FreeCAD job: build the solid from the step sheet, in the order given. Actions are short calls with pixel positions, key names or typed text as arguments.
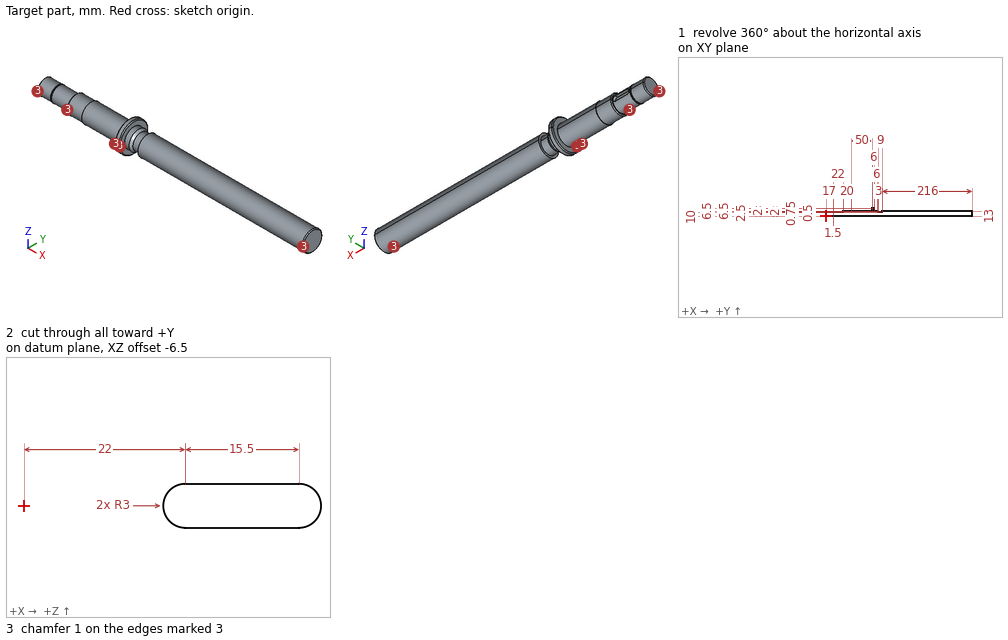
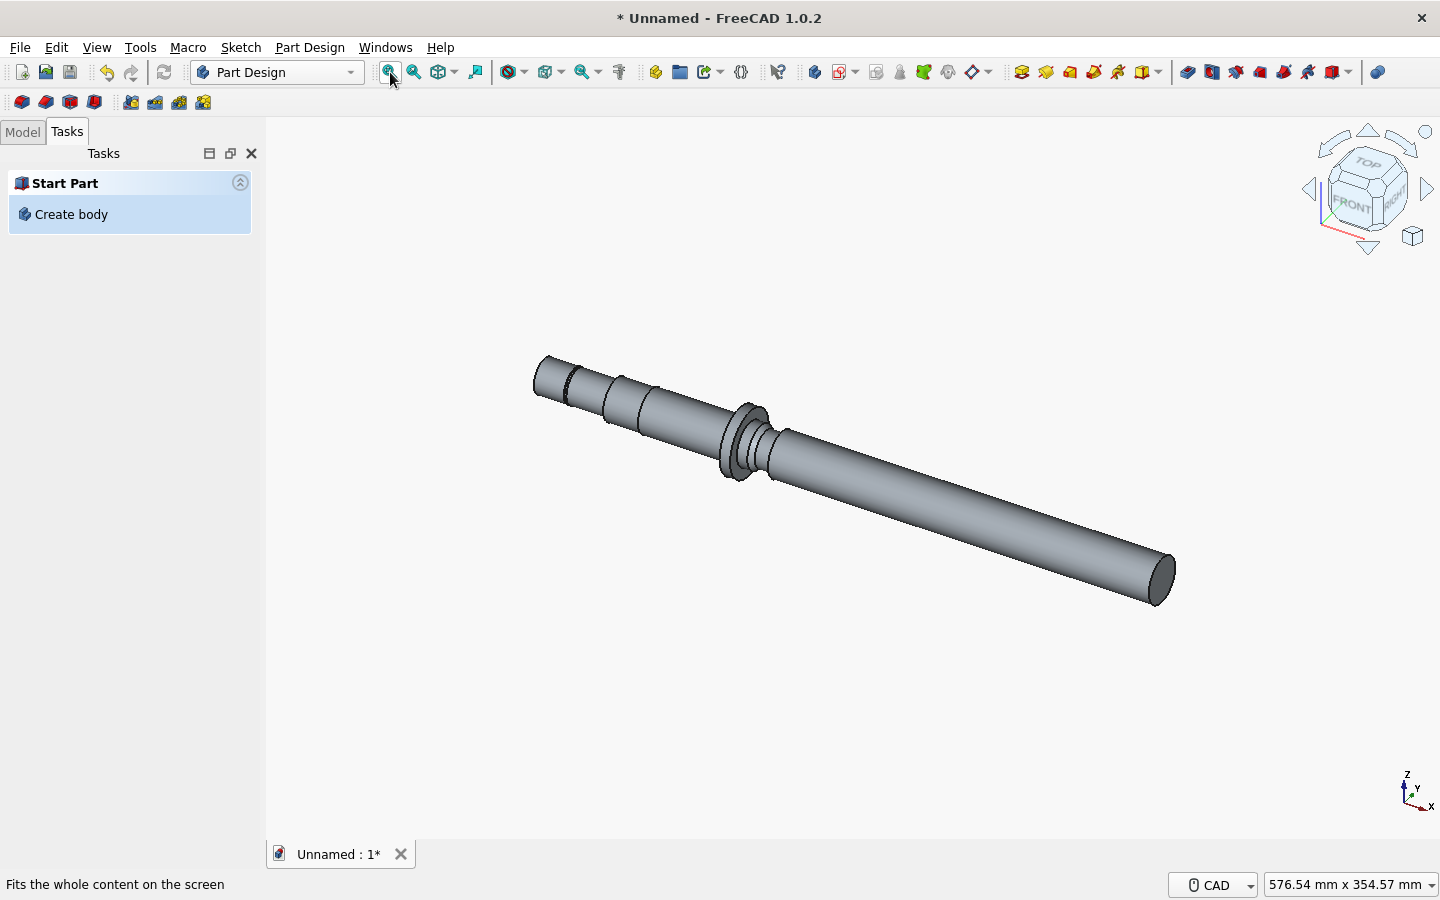
click(23, 131)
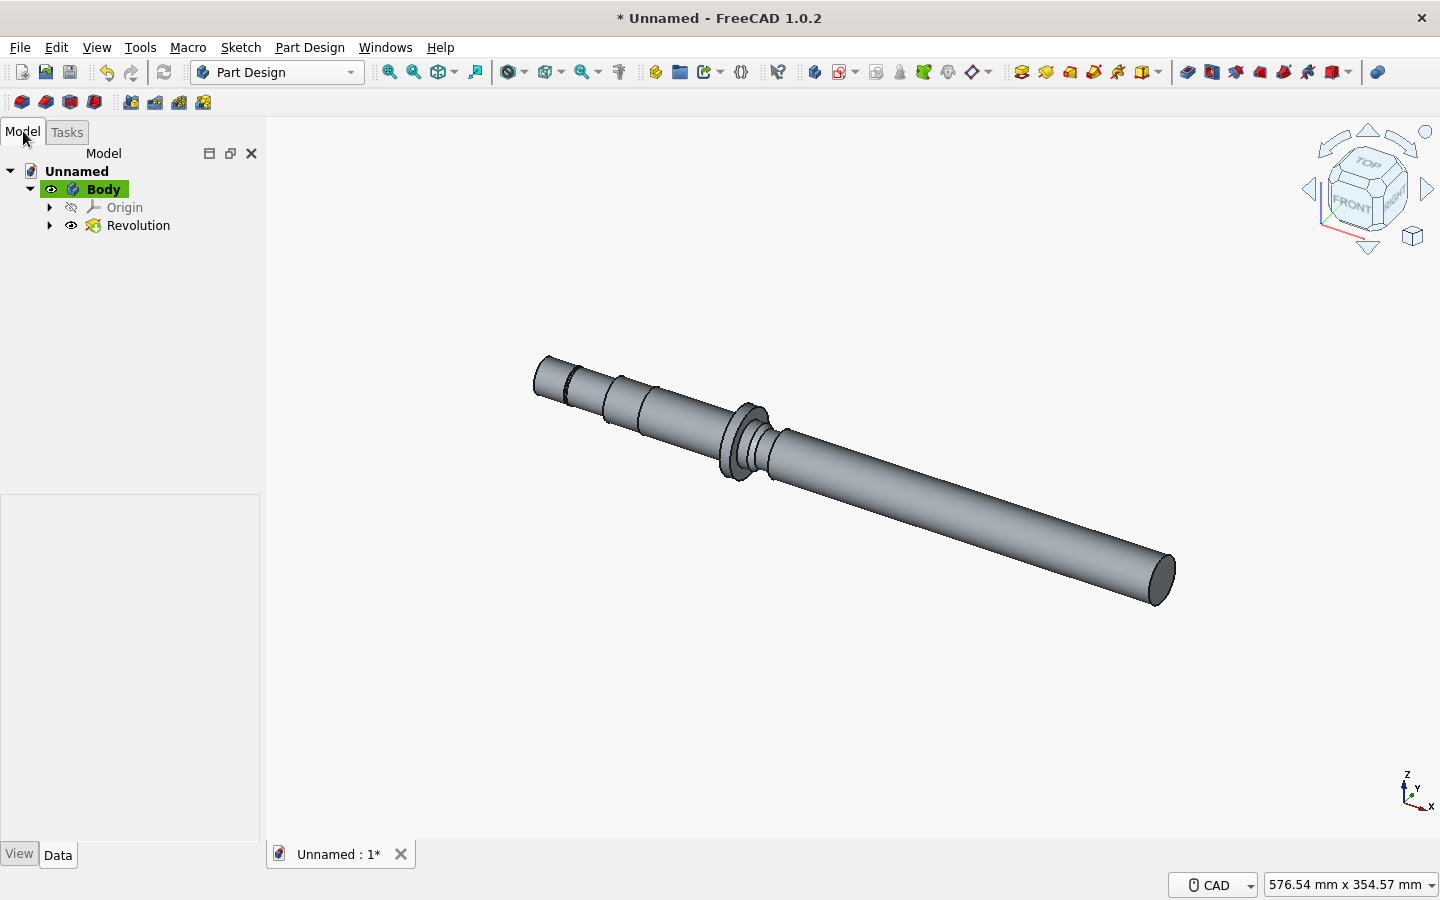
click(50, 207)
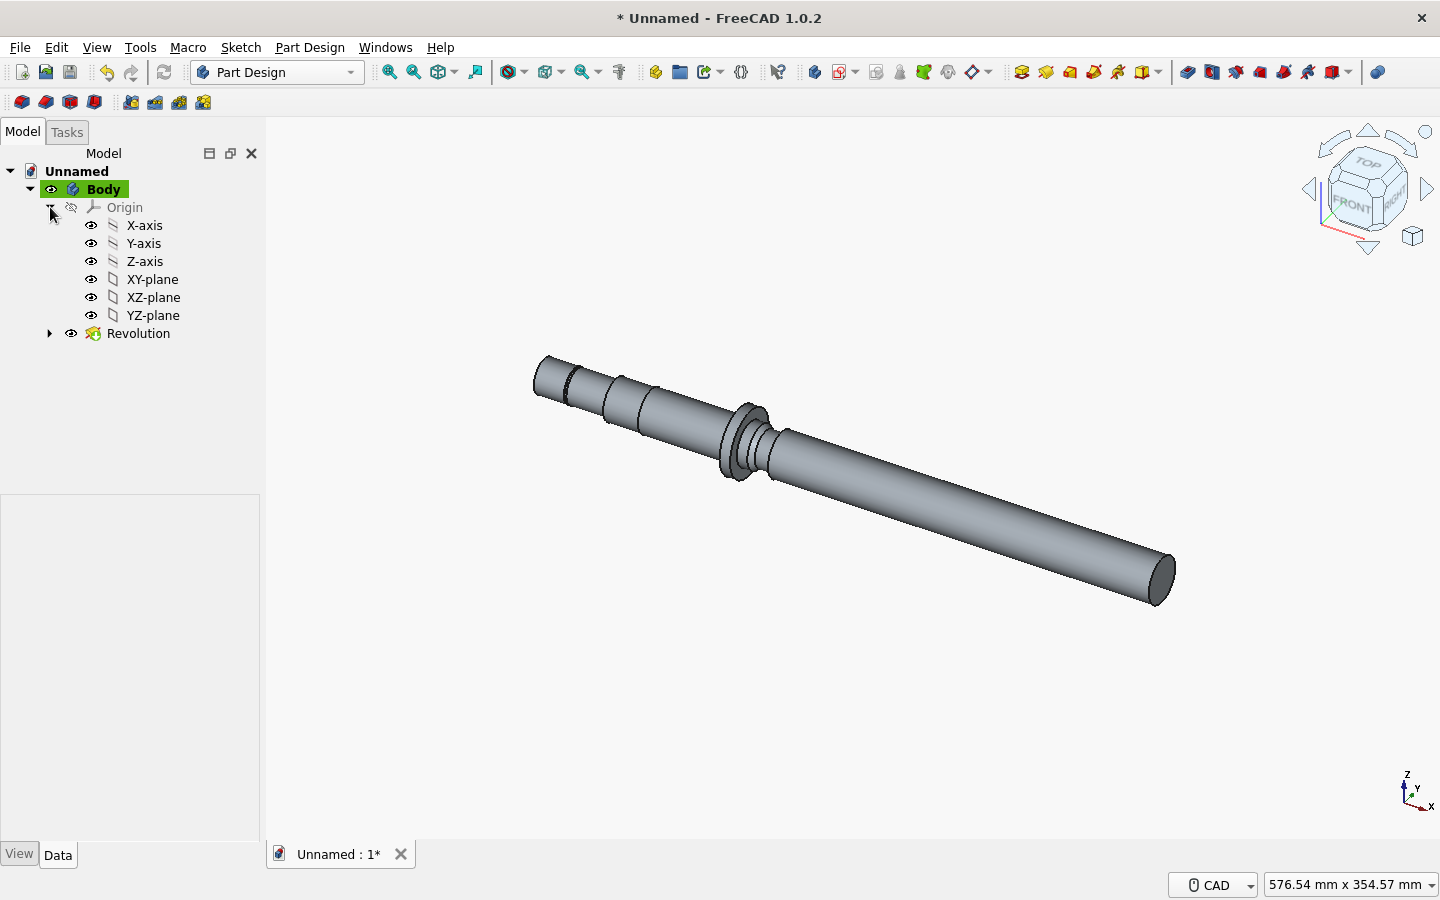
click(136, 297)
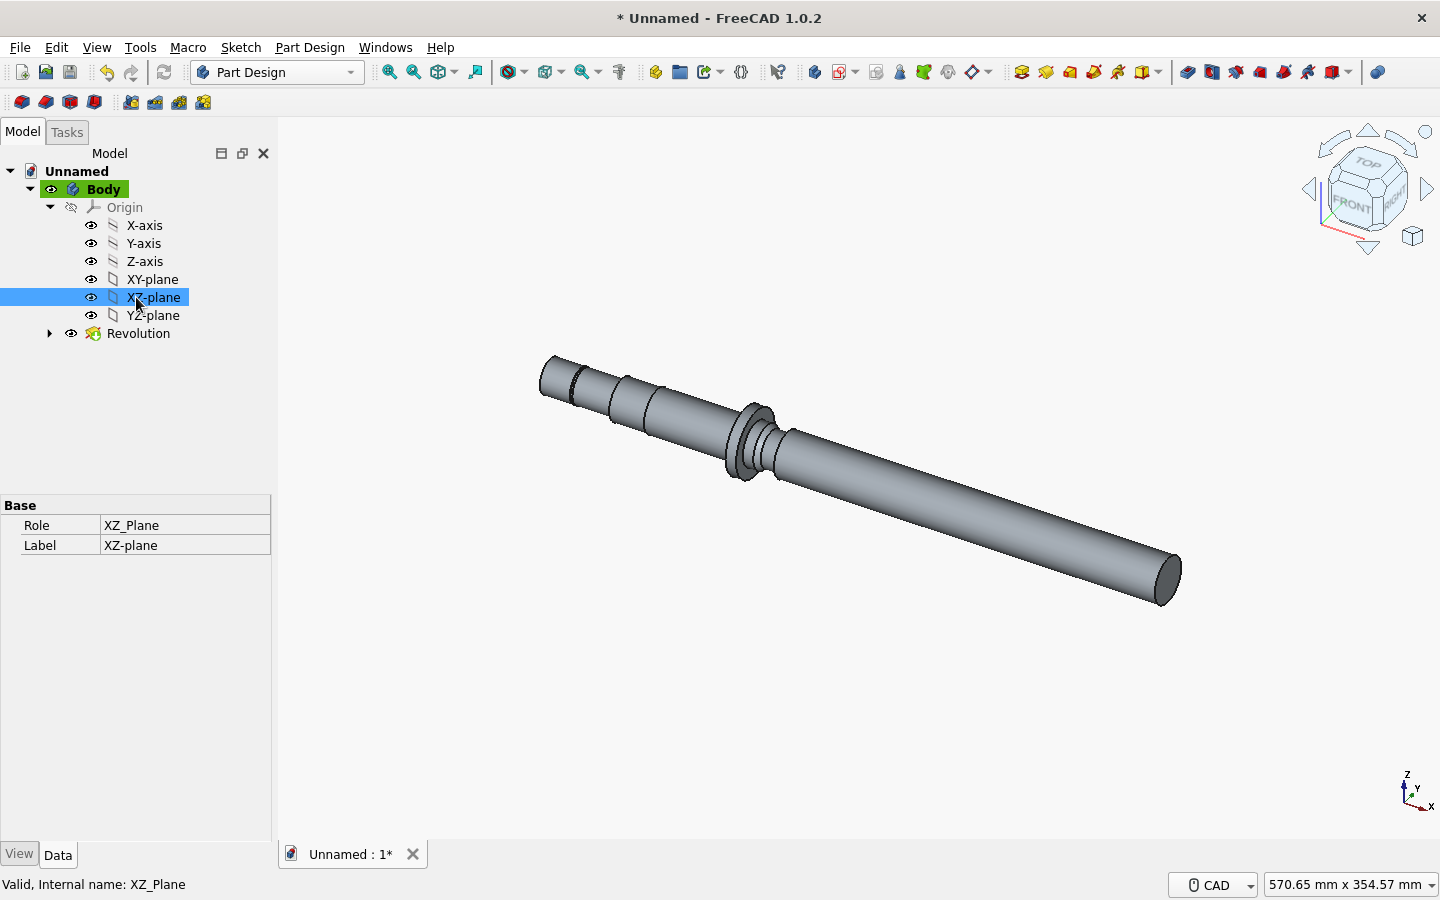
click(972, 72)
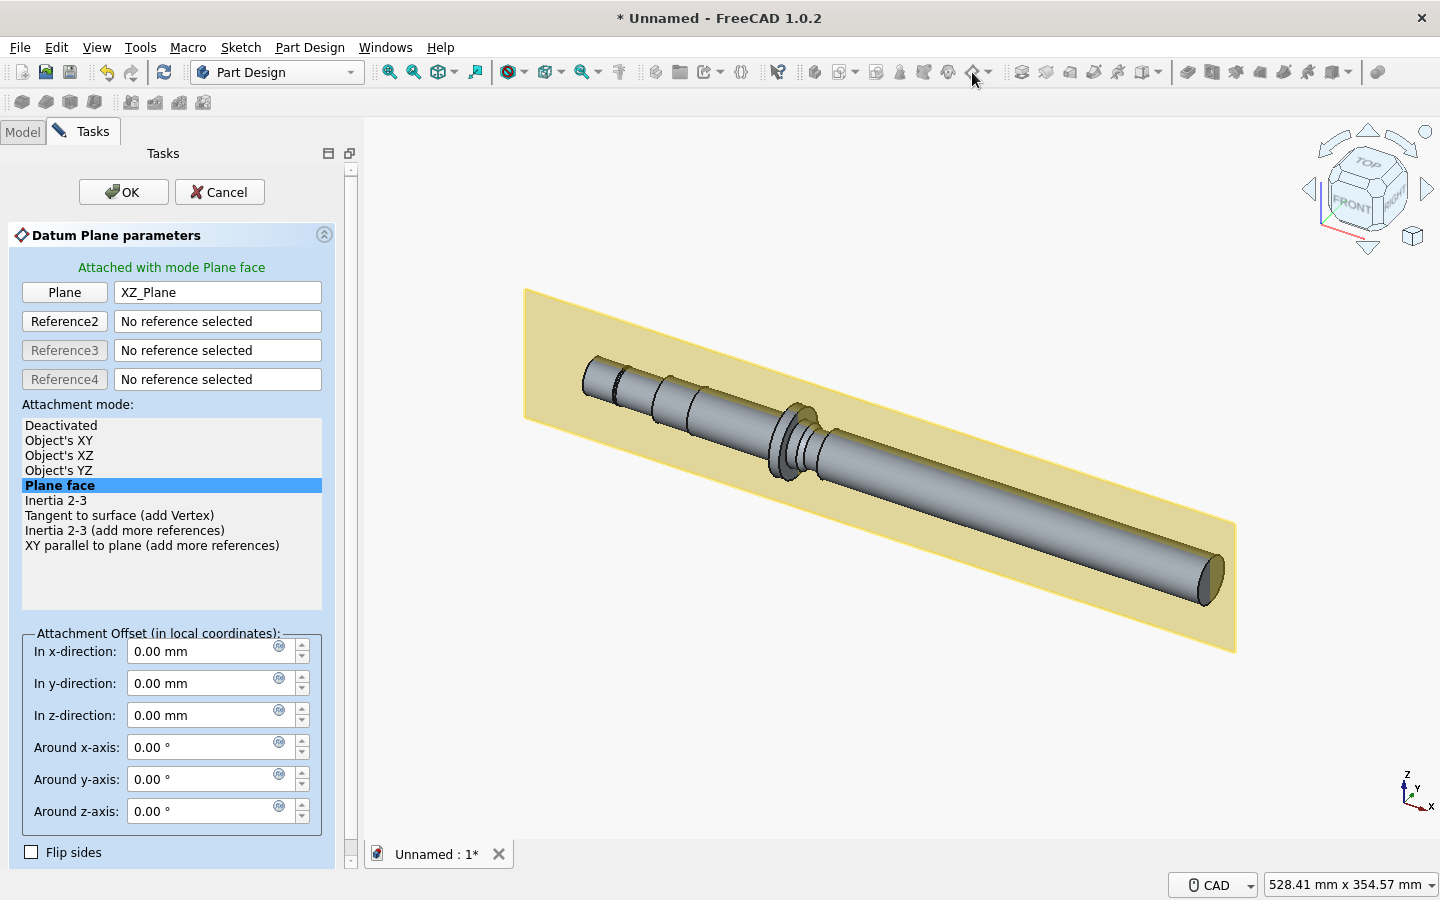
triple_click(210, 715)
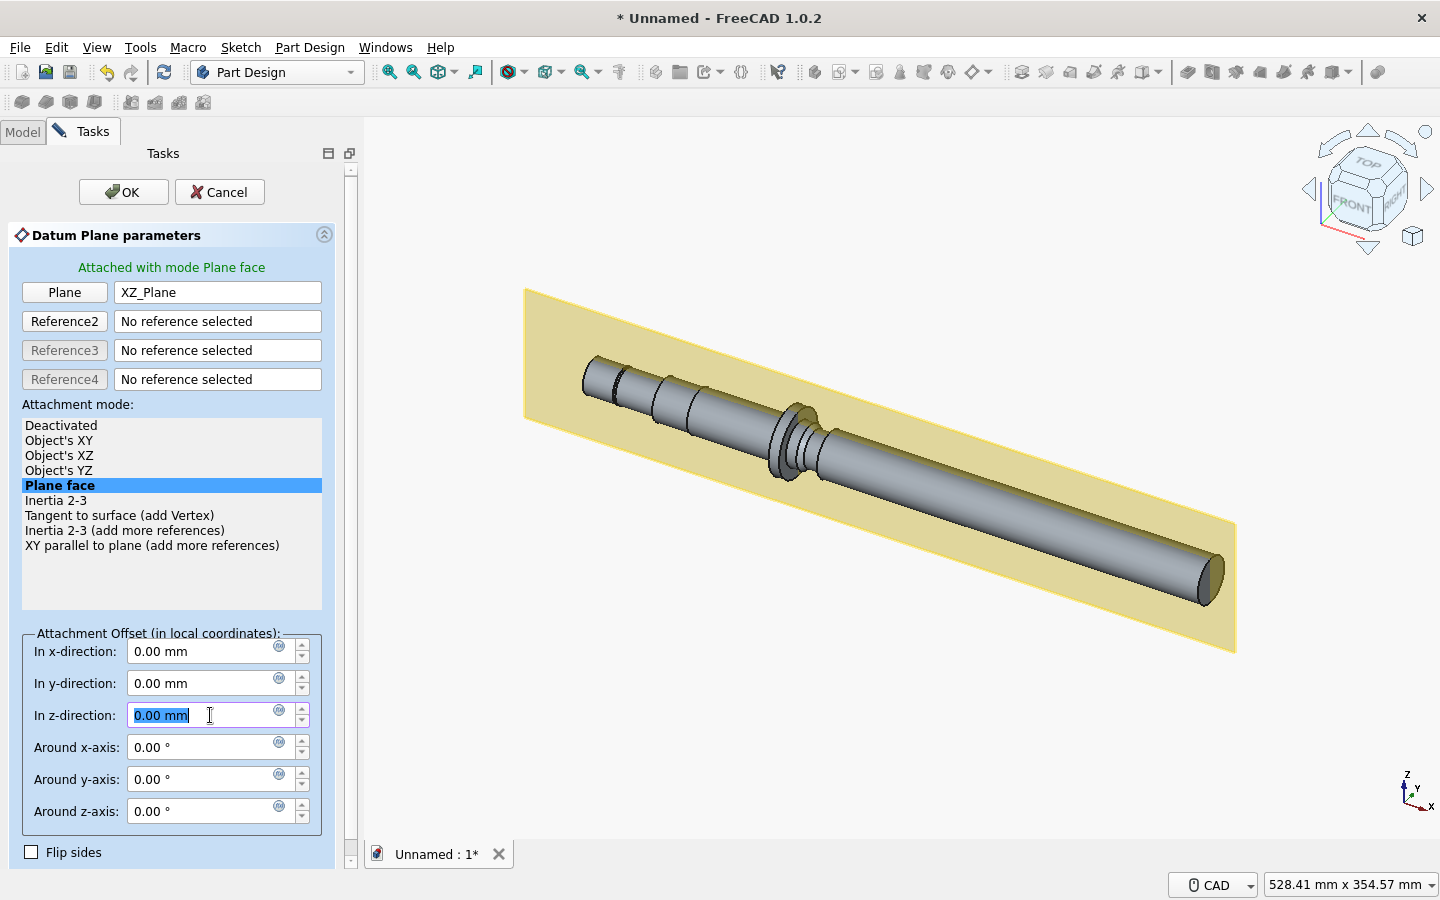
text(-6.5)
key(Tab)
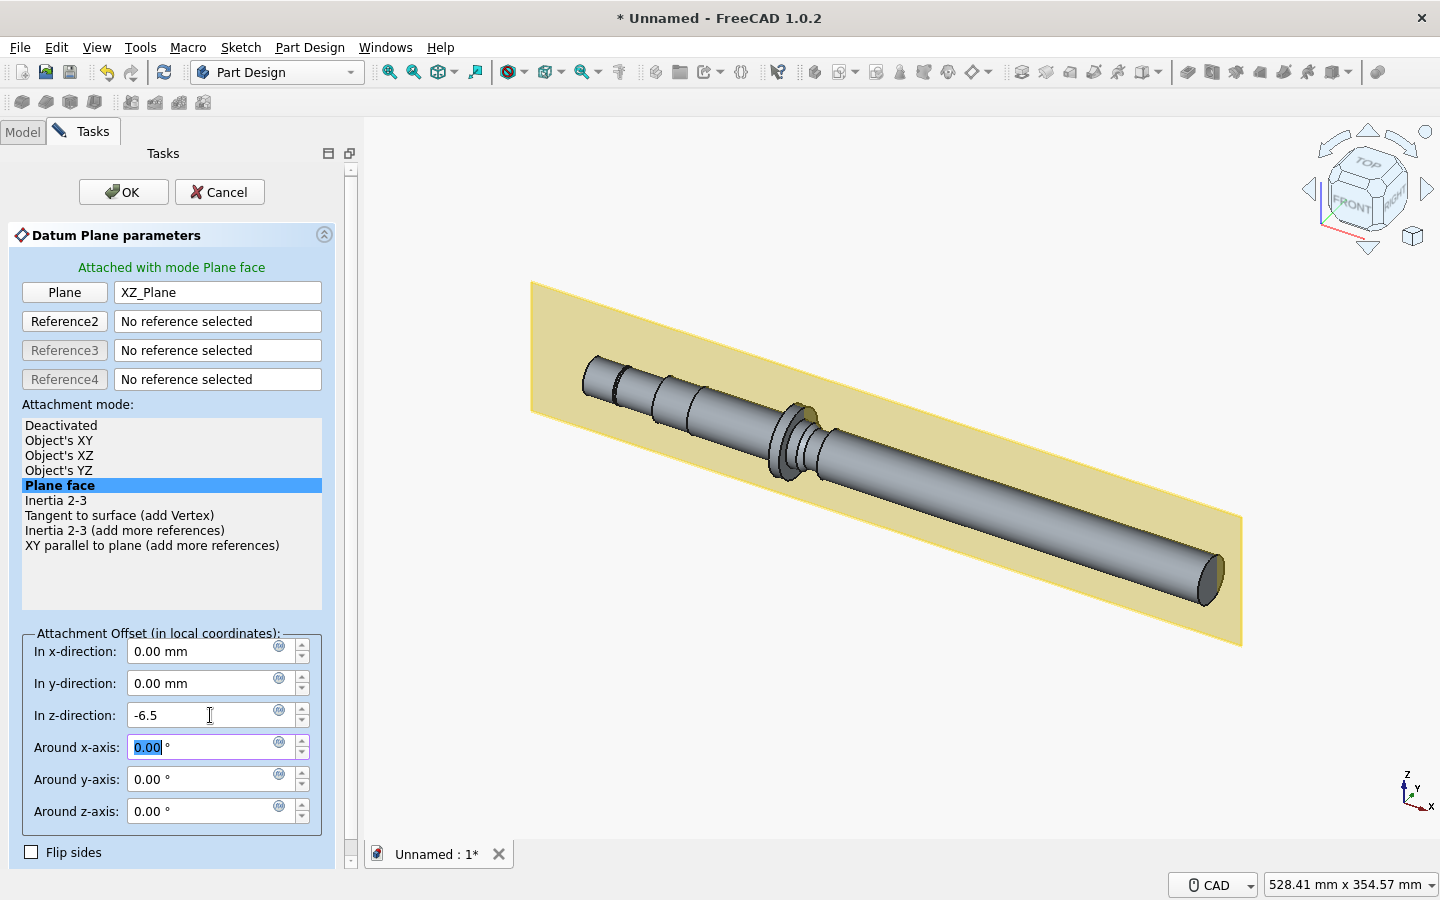
click(124, 192)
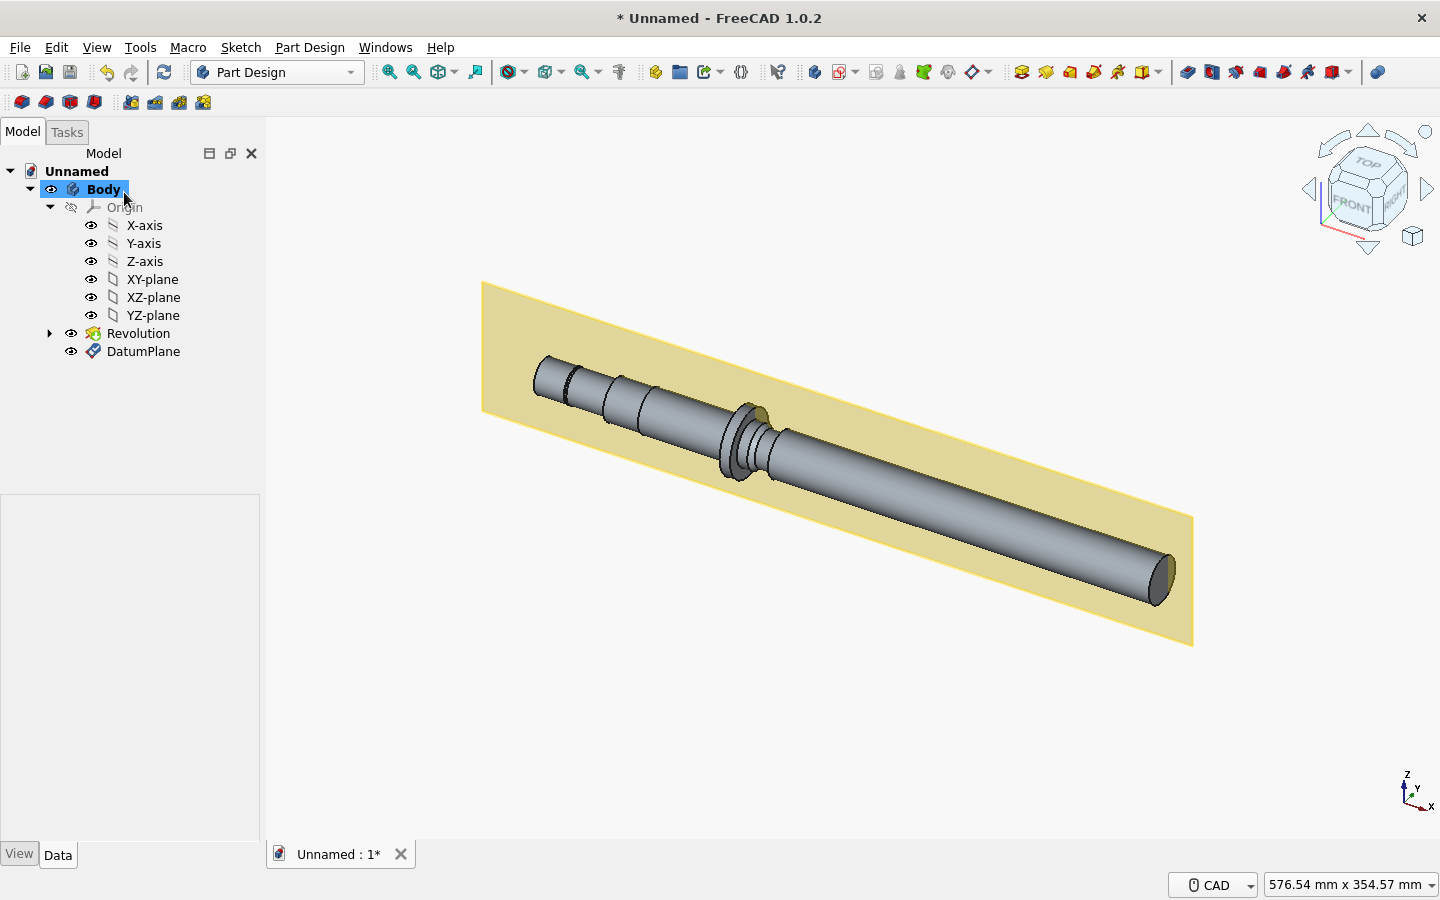
click(116, 351)